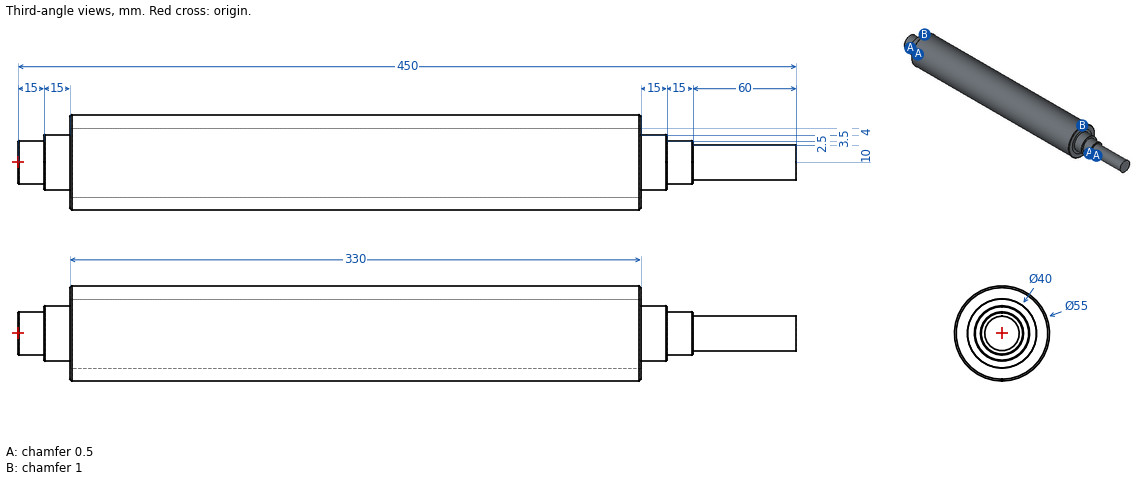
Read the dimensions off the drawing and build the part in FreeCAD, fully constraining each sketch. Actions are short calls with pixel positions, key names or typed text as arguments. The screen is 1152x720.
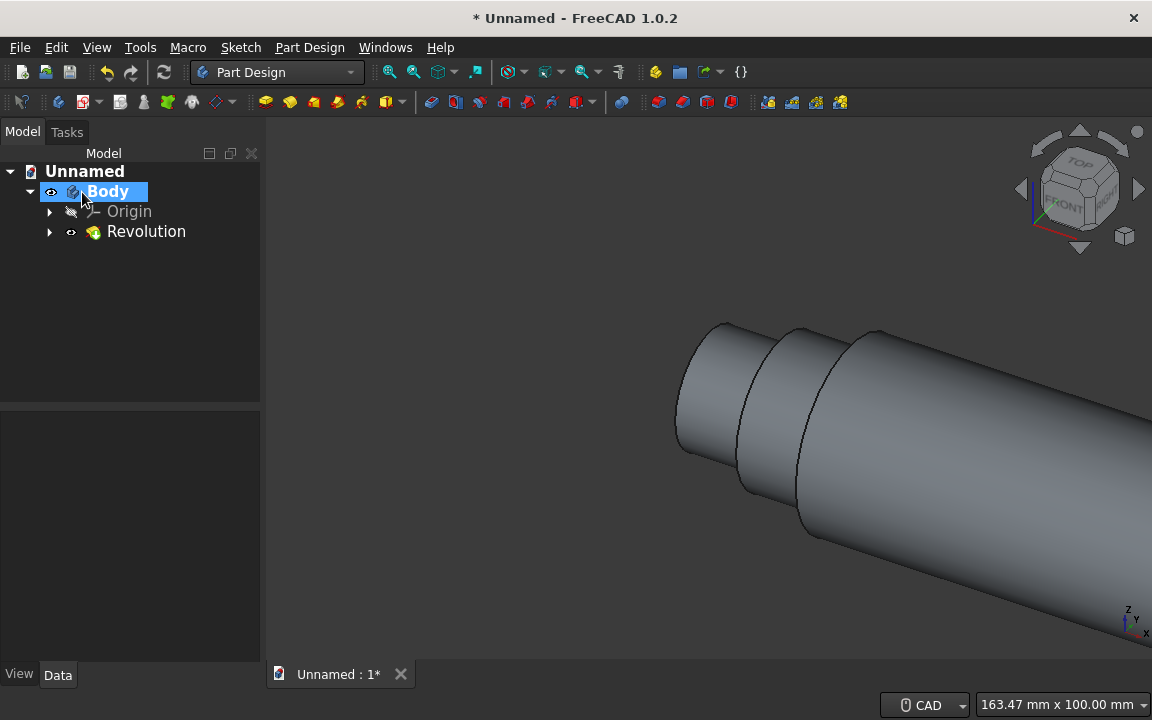
key(v)
key(f)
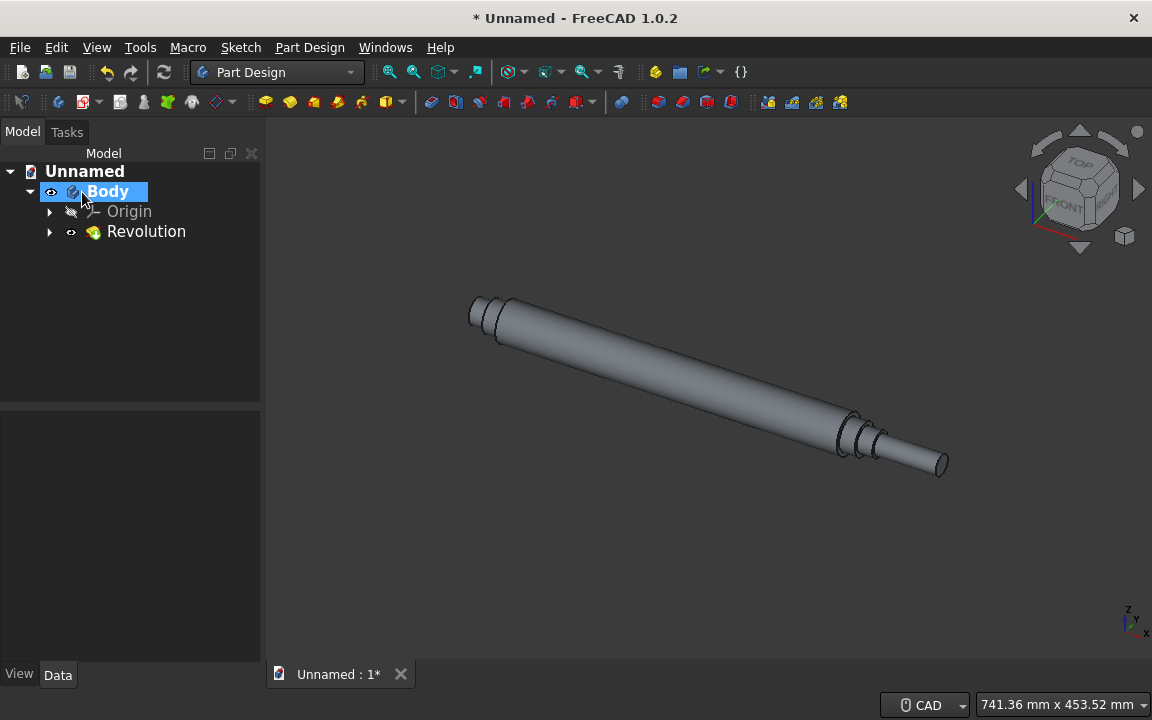
click(482, 325)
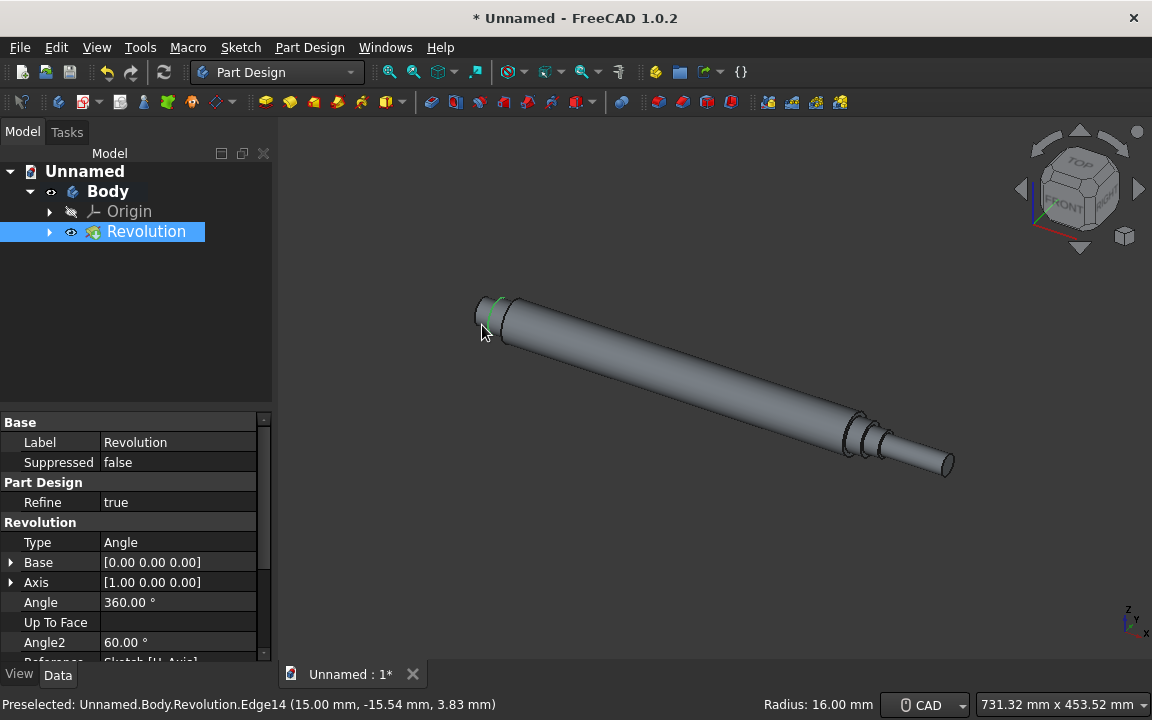
click(861, 448, ctrl)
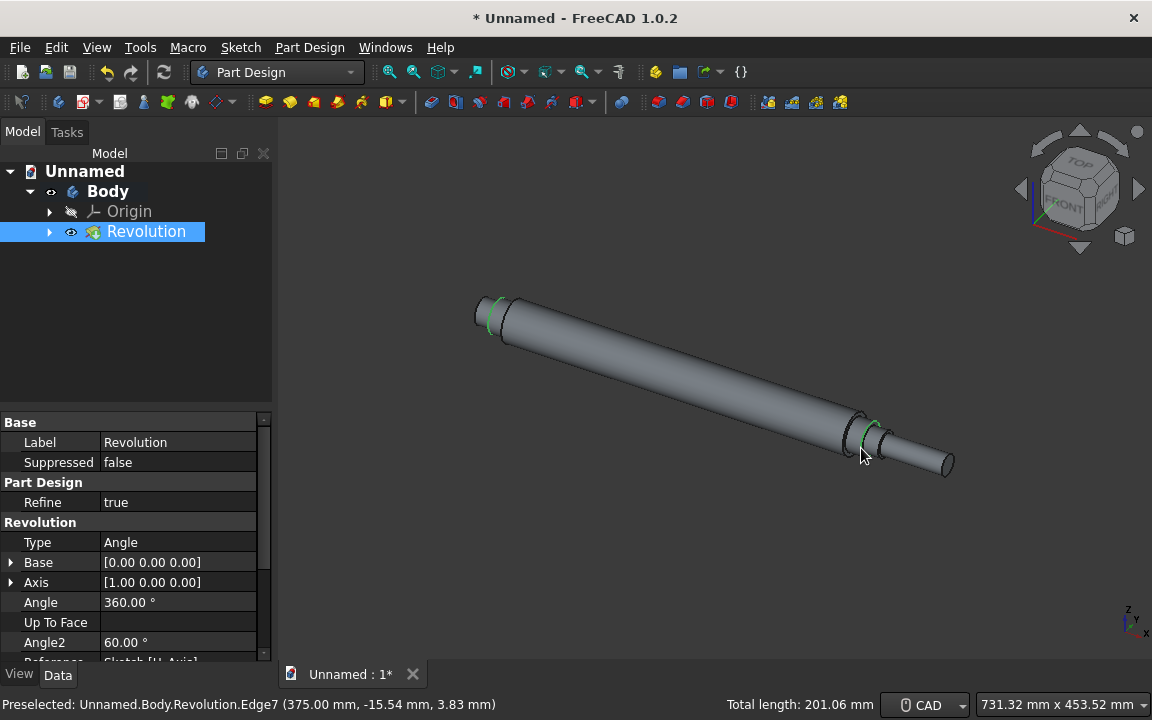
click(878, 451, ctrl)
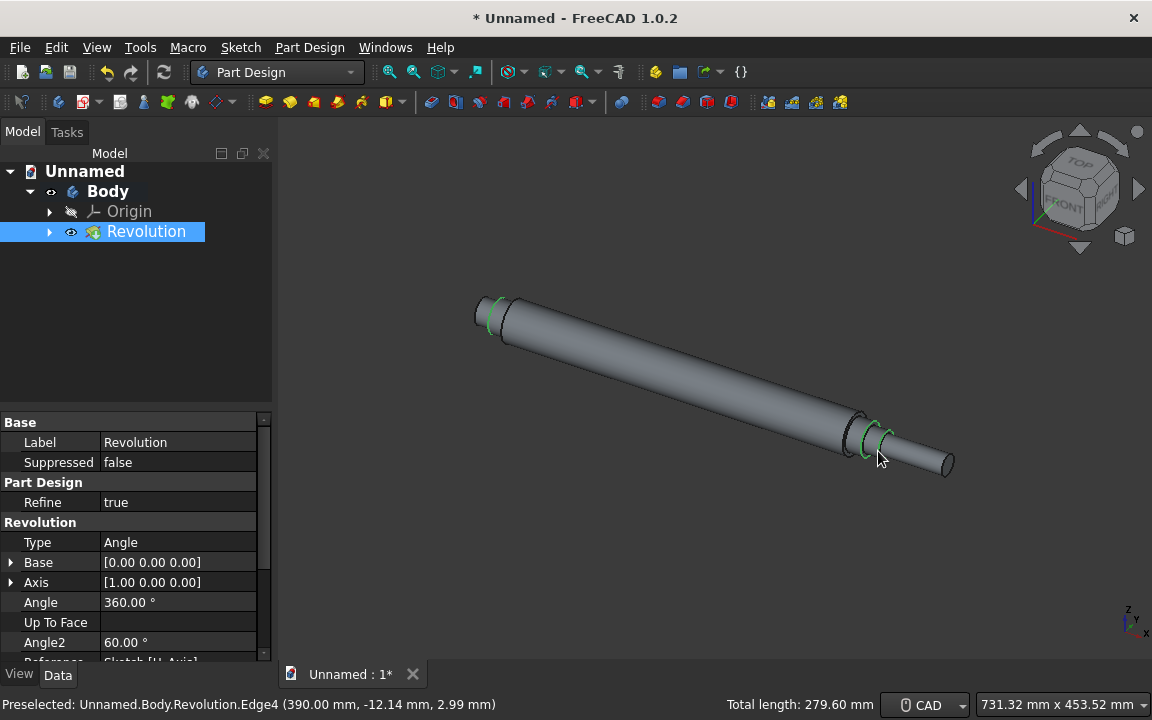
click(475, 317, ctrl)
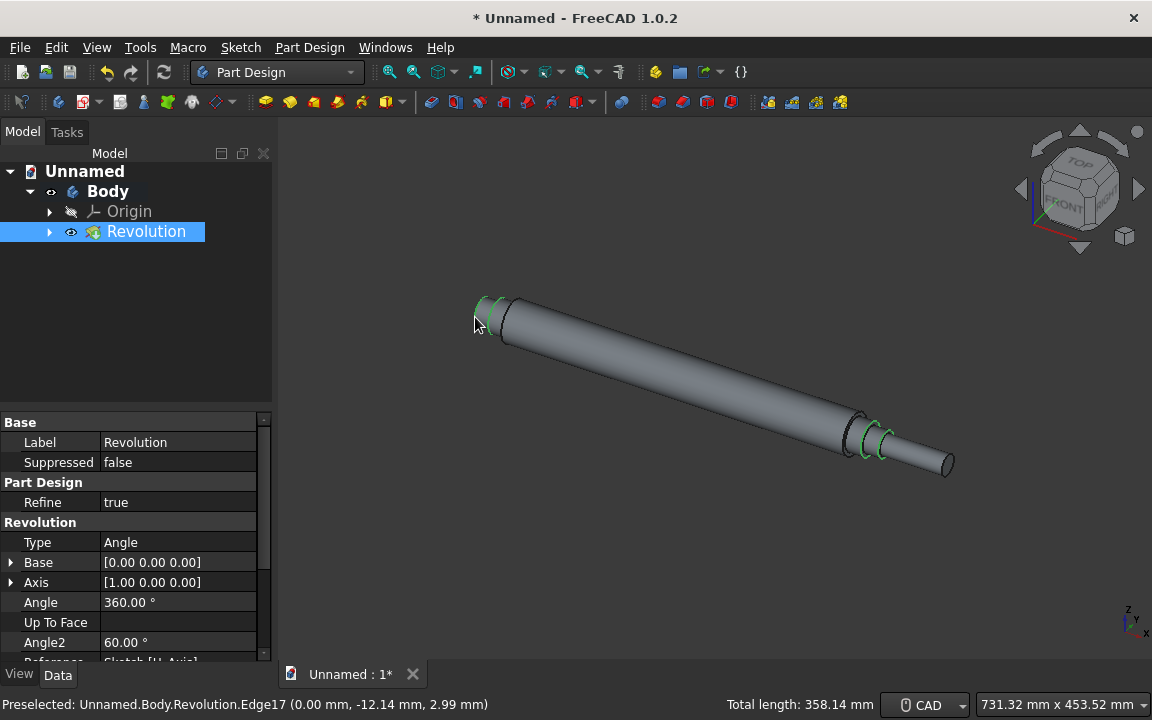
click(684, 102)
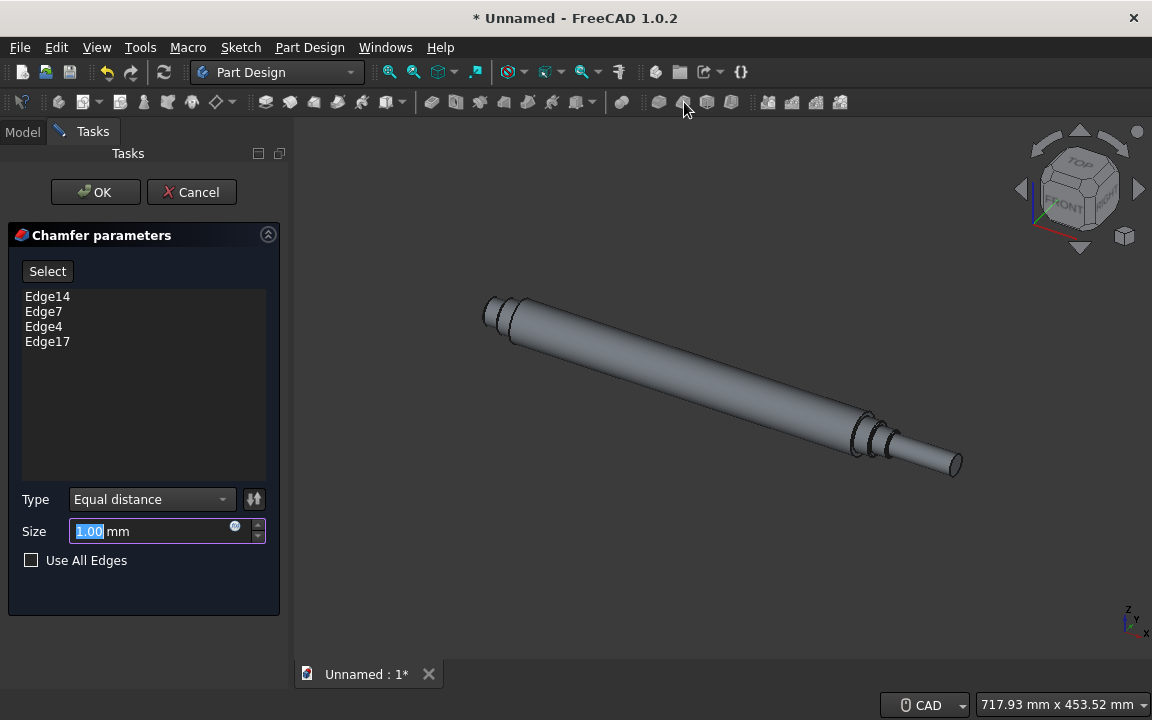
text(0.5)
key(Tab)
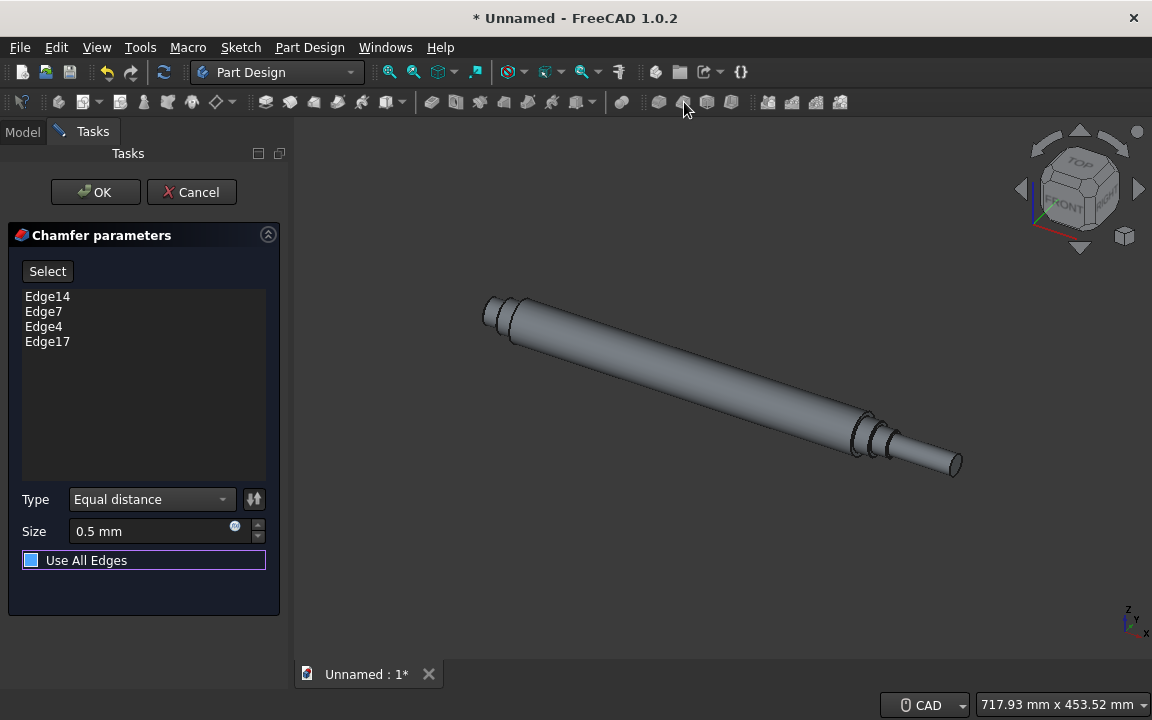
click(96, 192)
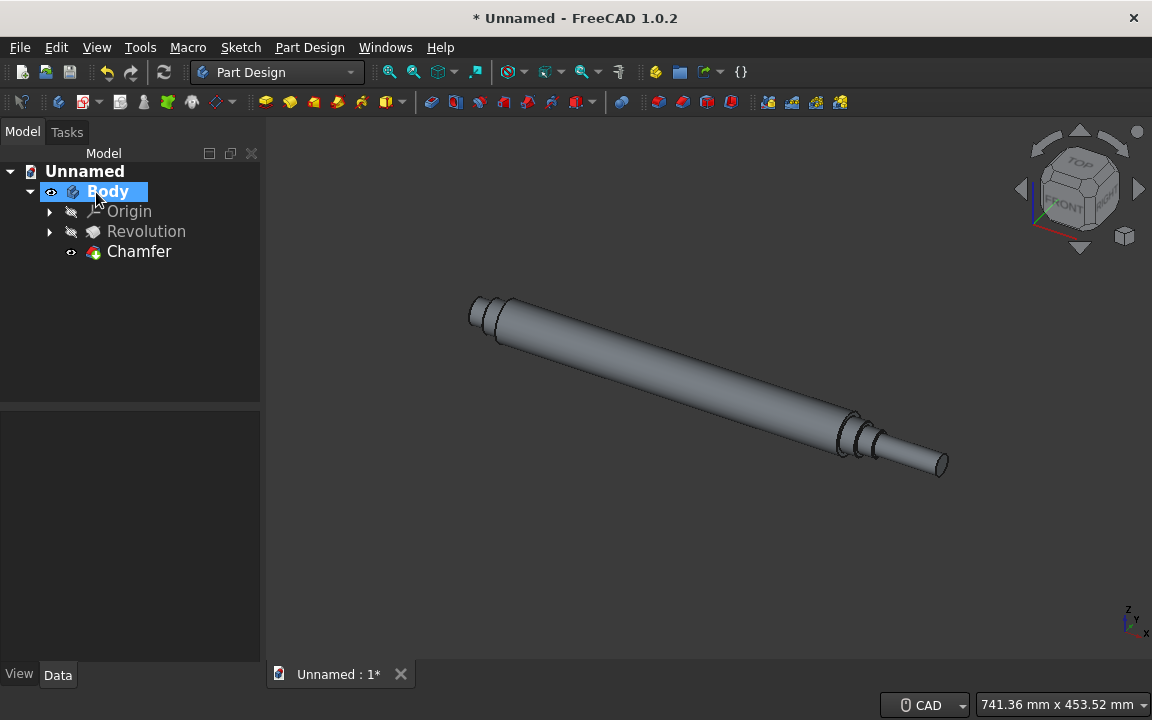
click(60, 102)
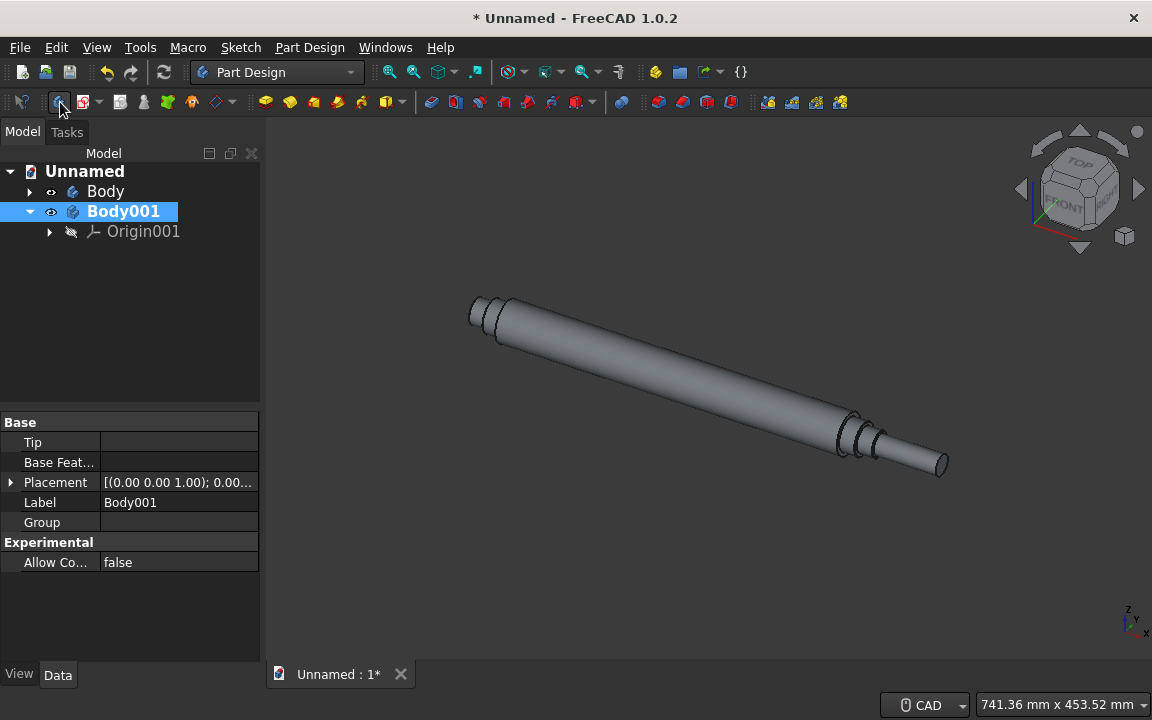
click(50, 232)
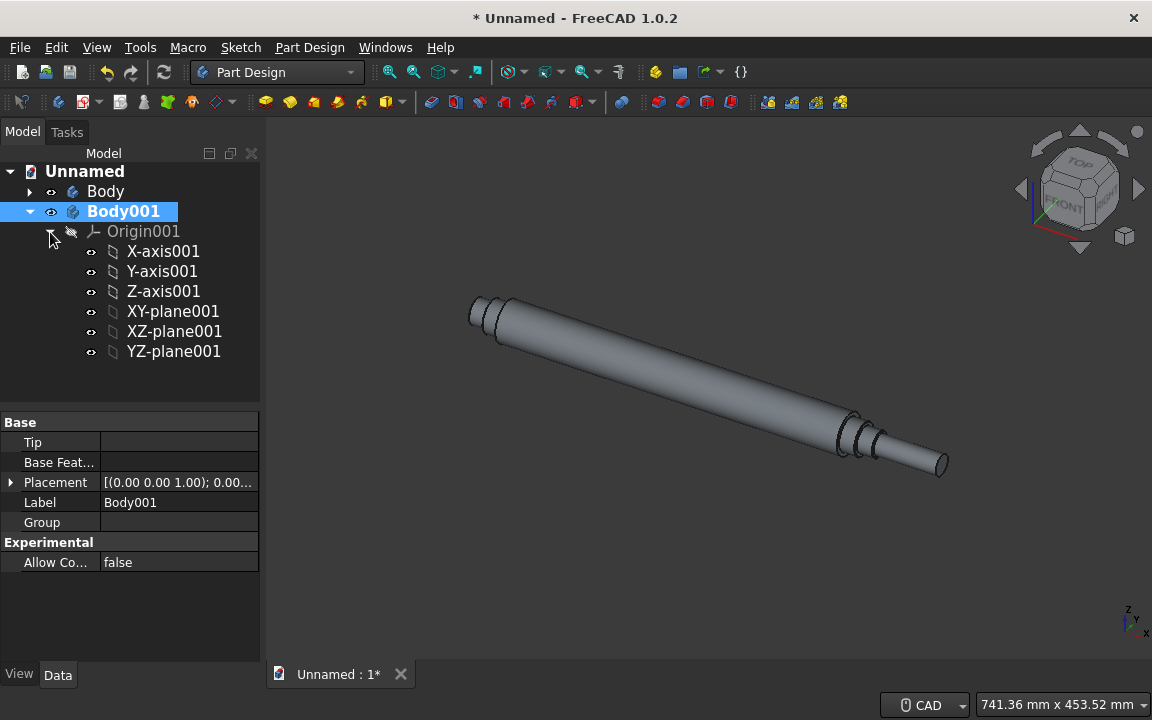
click(136, 352)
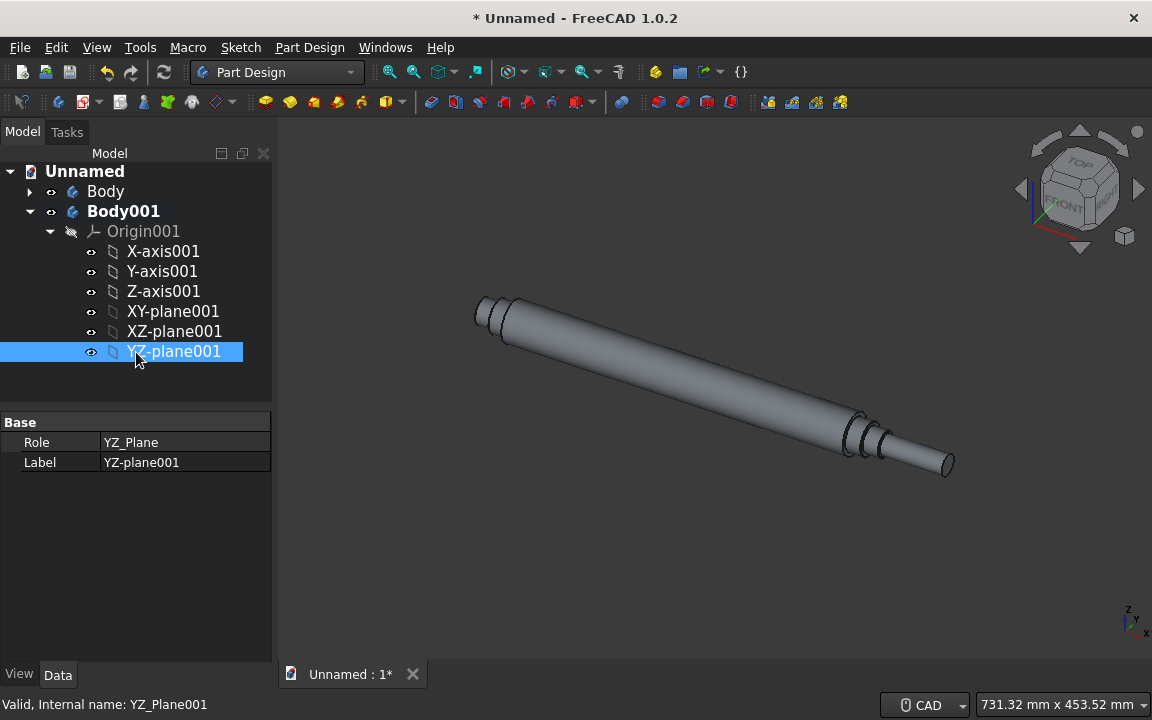
click(216, 102)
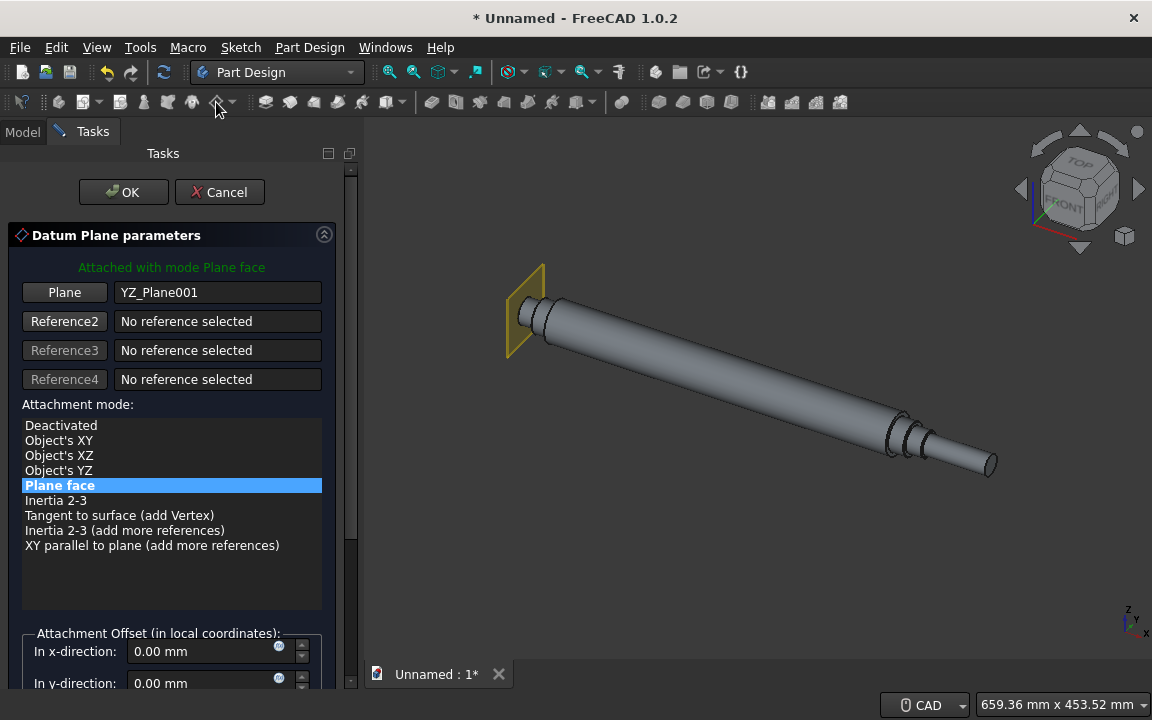
scroll(351, 426, down, 2)